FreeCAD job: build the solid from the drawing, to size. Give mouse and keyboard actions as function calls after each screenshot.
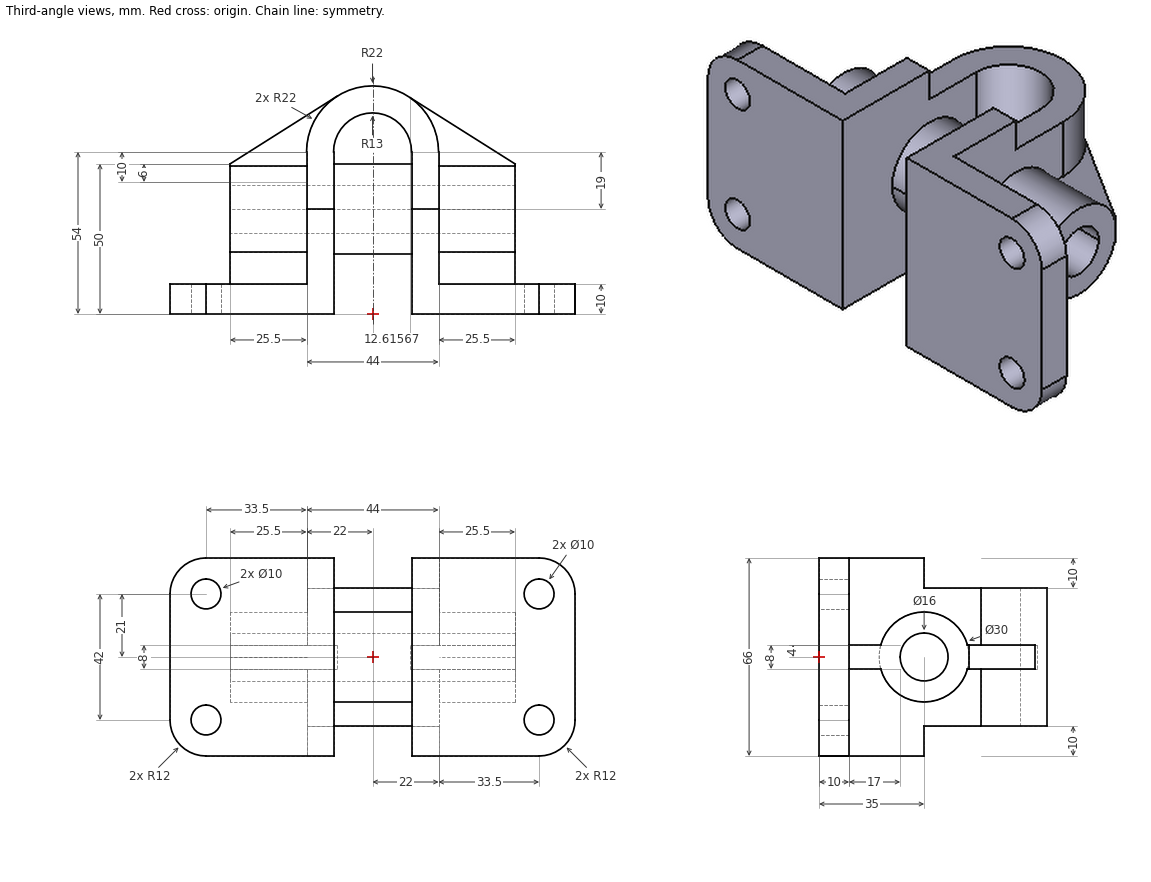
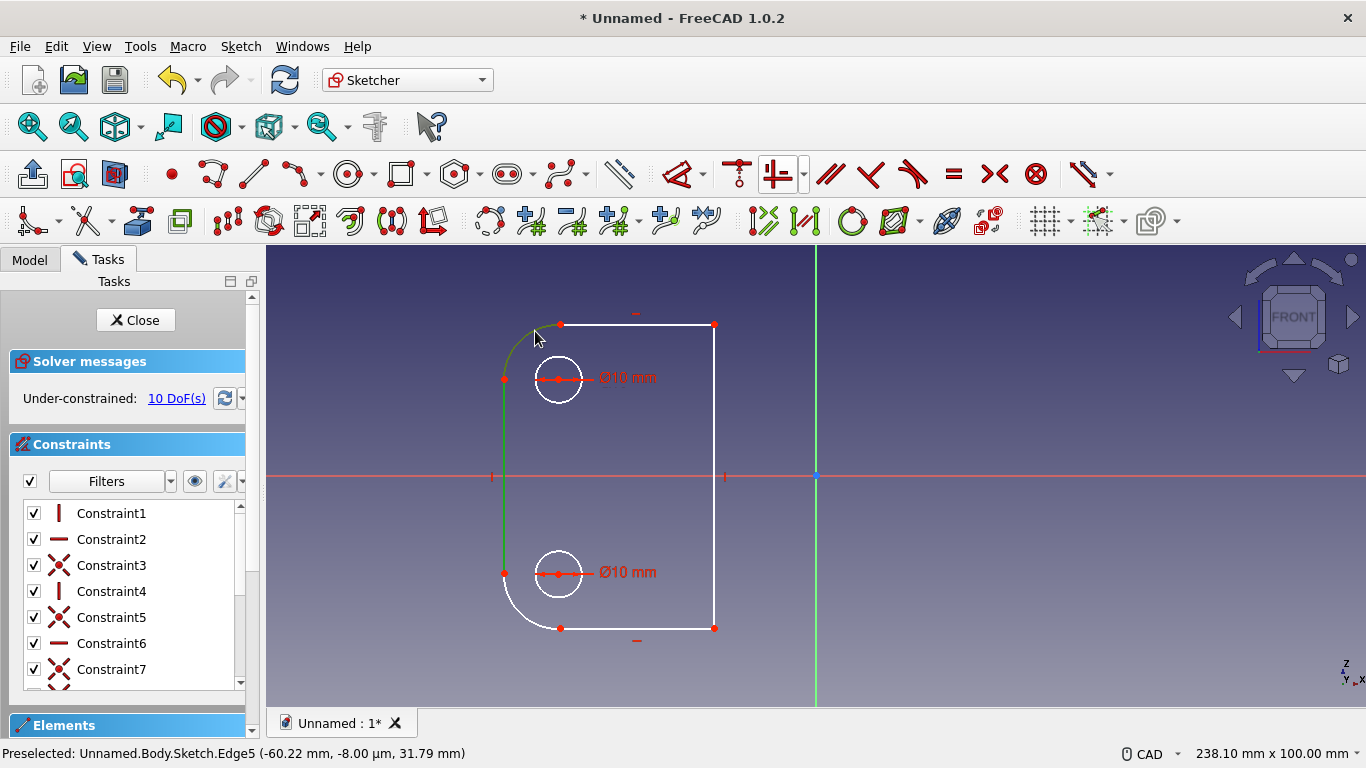
click(913, 174)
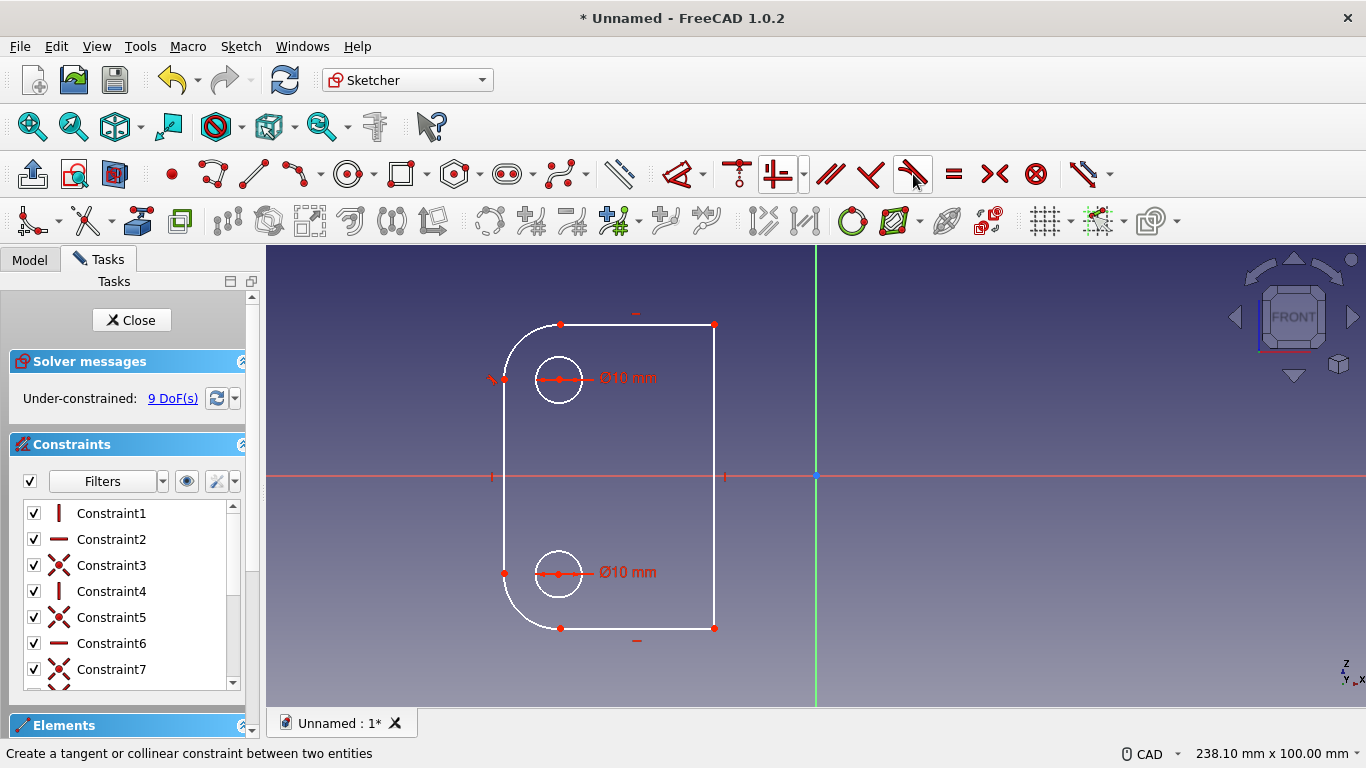
click(504, 516)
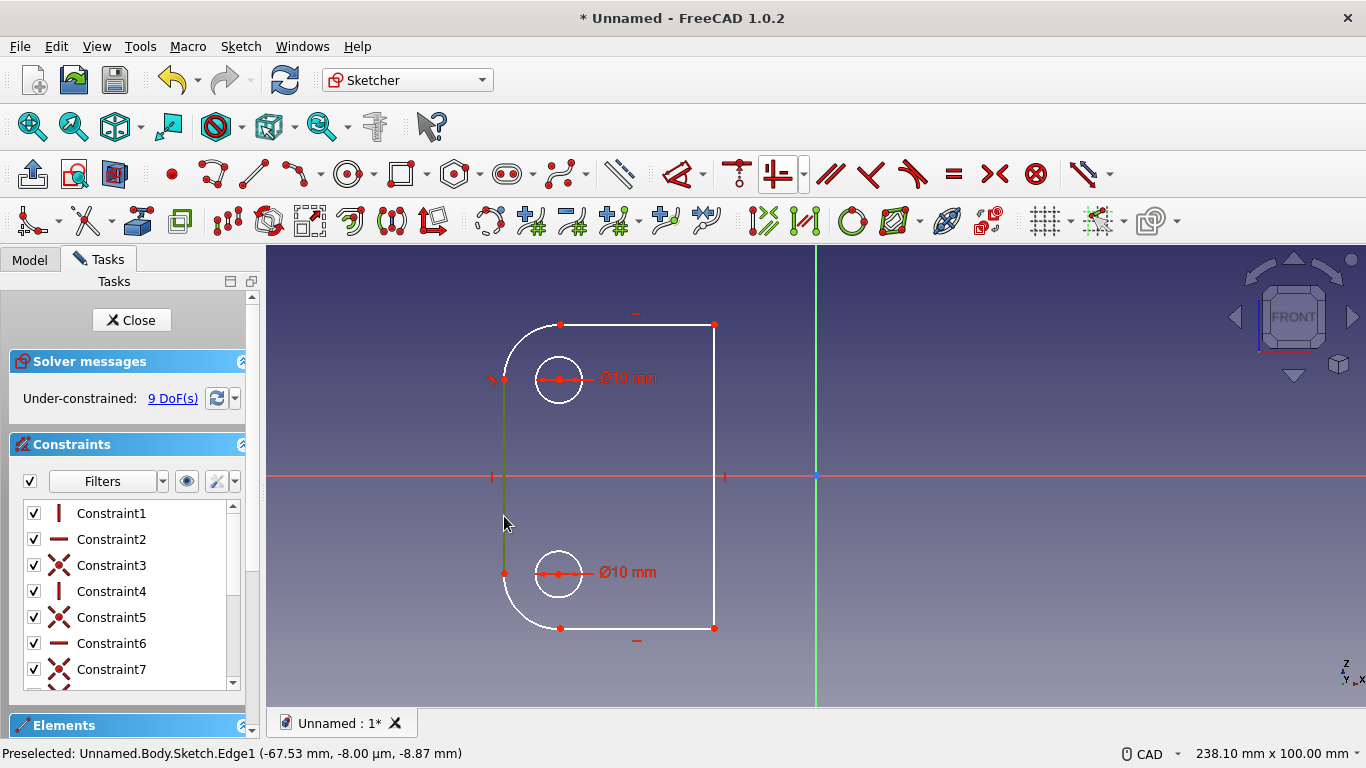
click(510, 599)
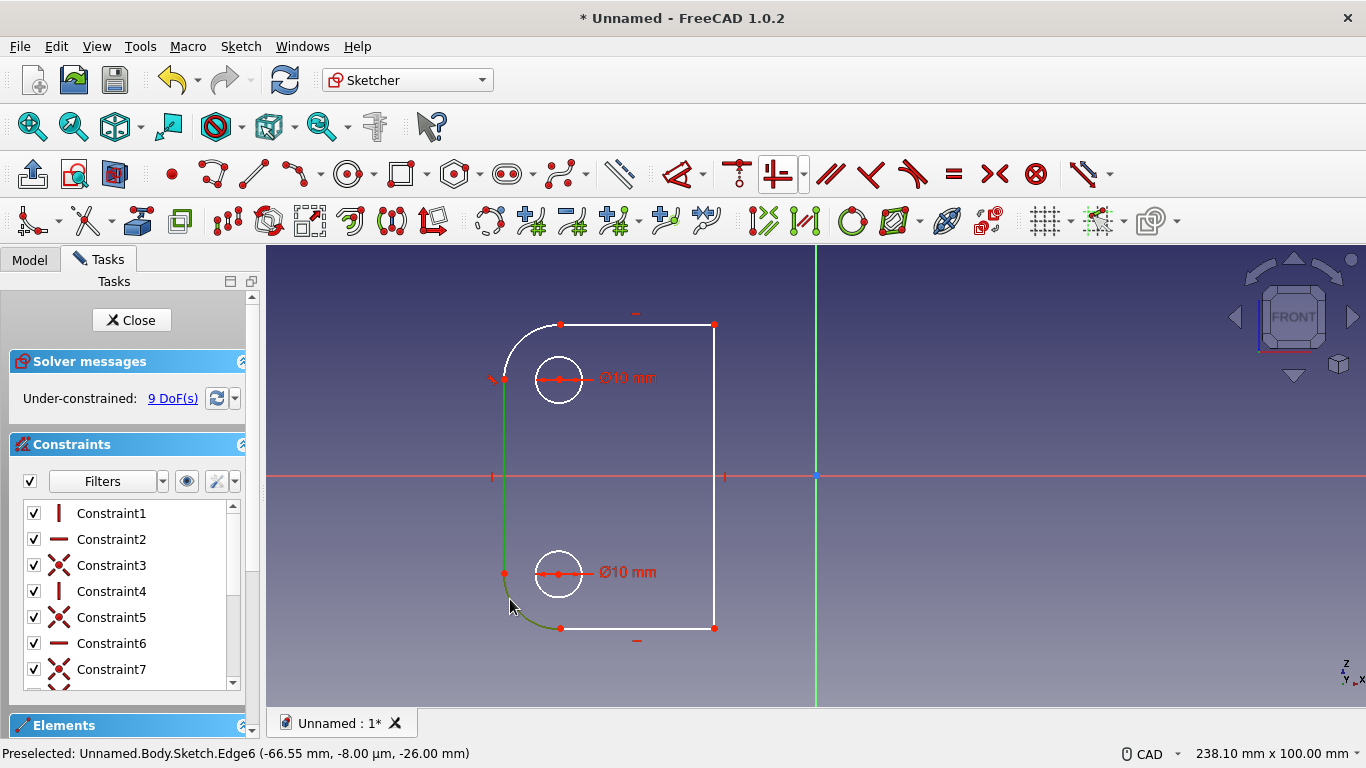
click(913, 174)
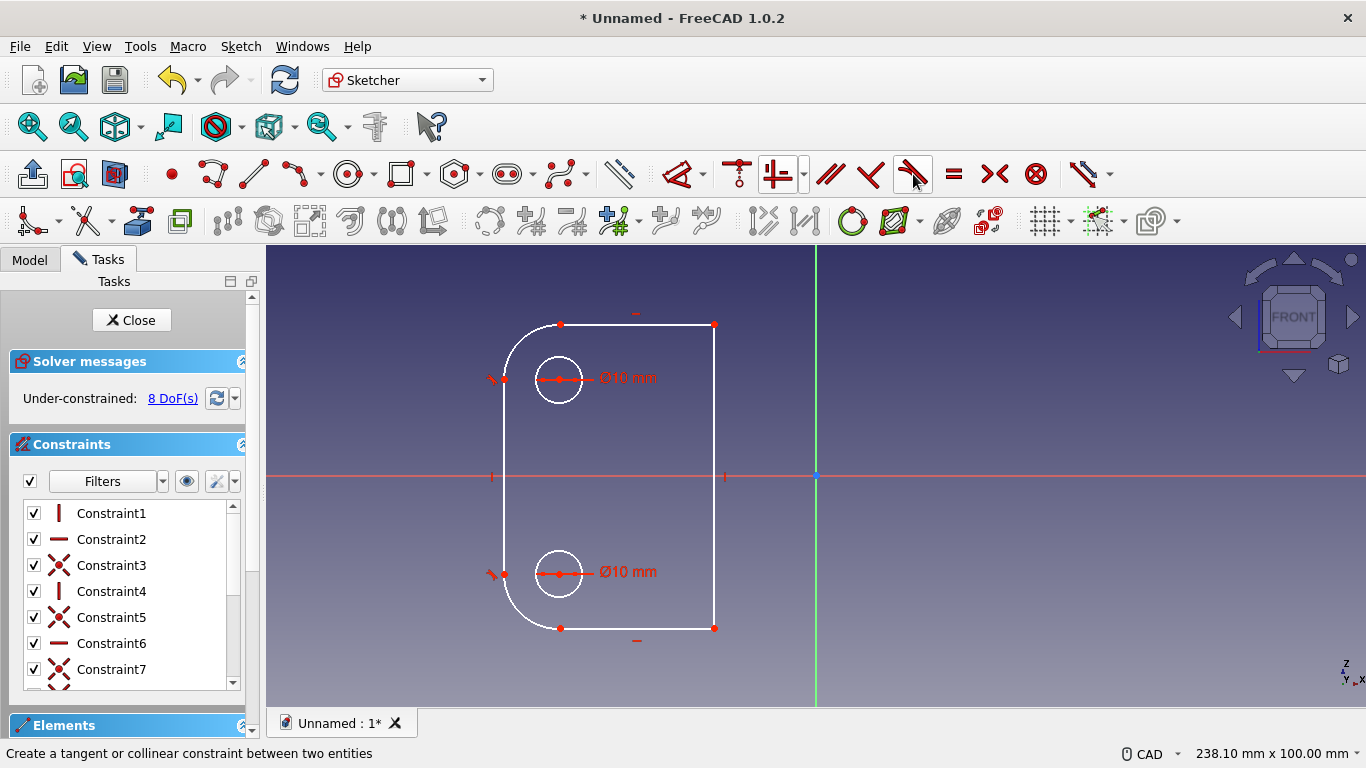
click(606, 325)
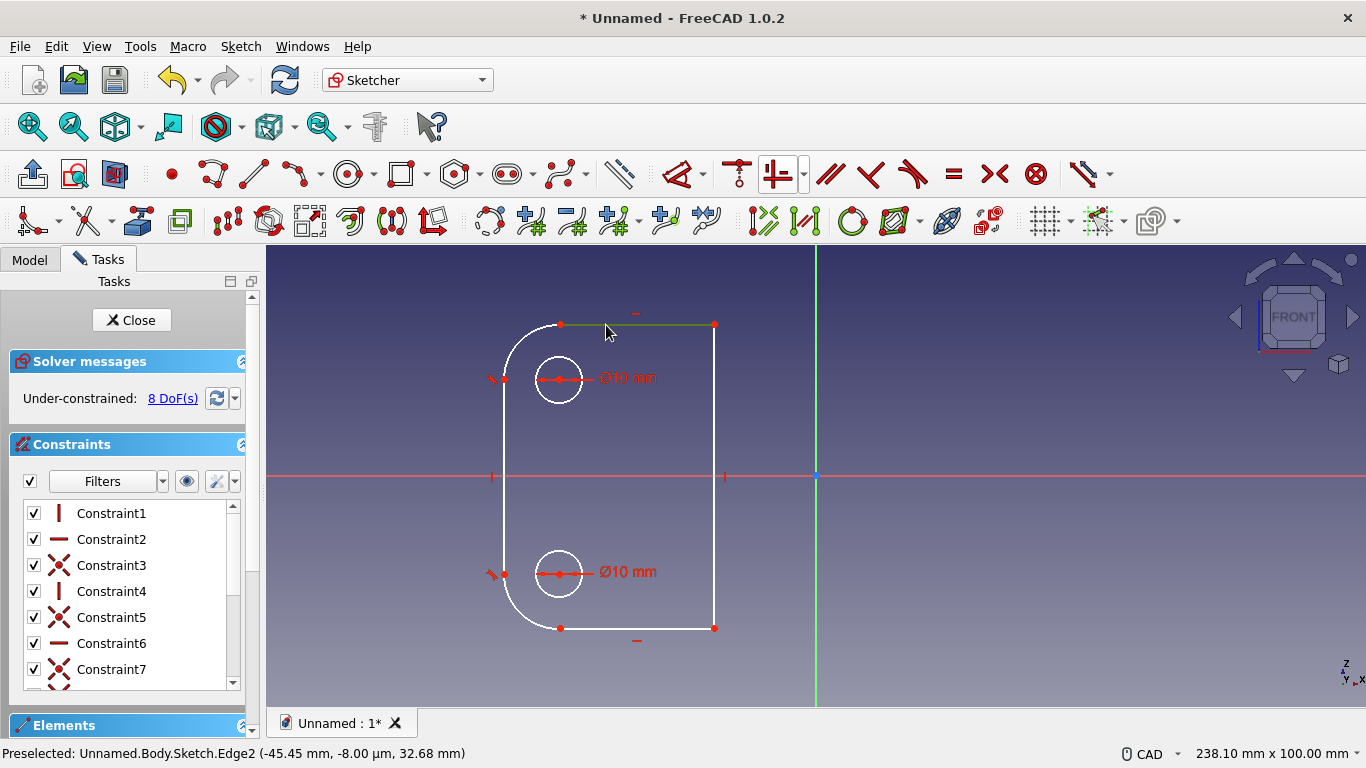
click(535, 331)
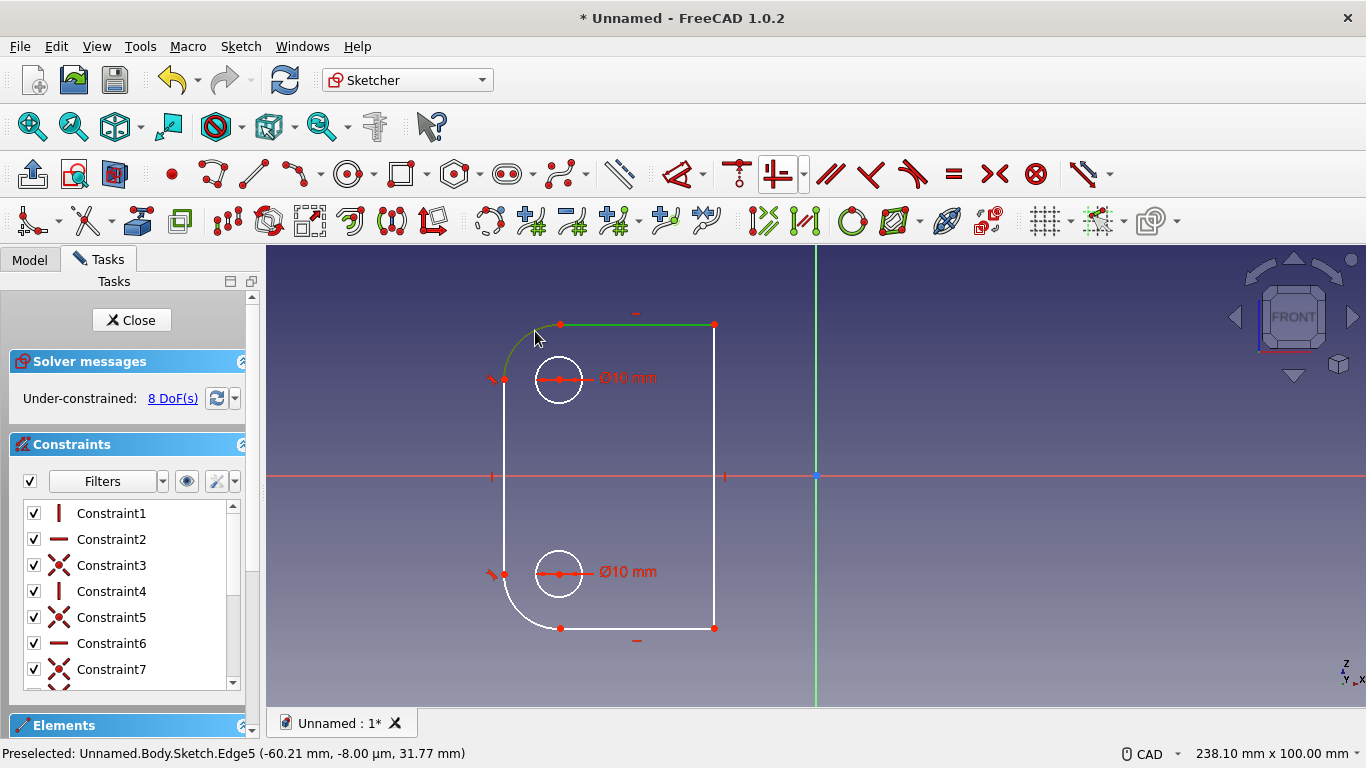
click(913, 174)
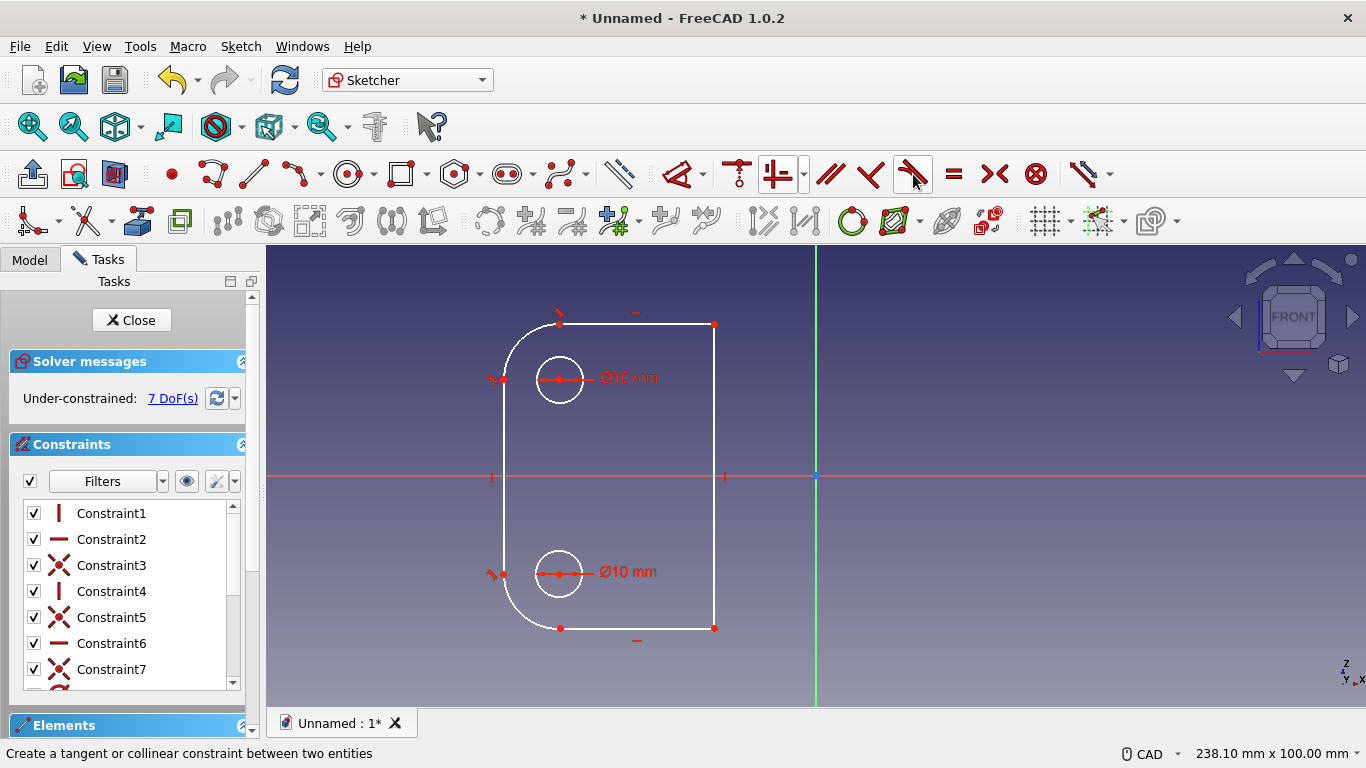
click(668, 629)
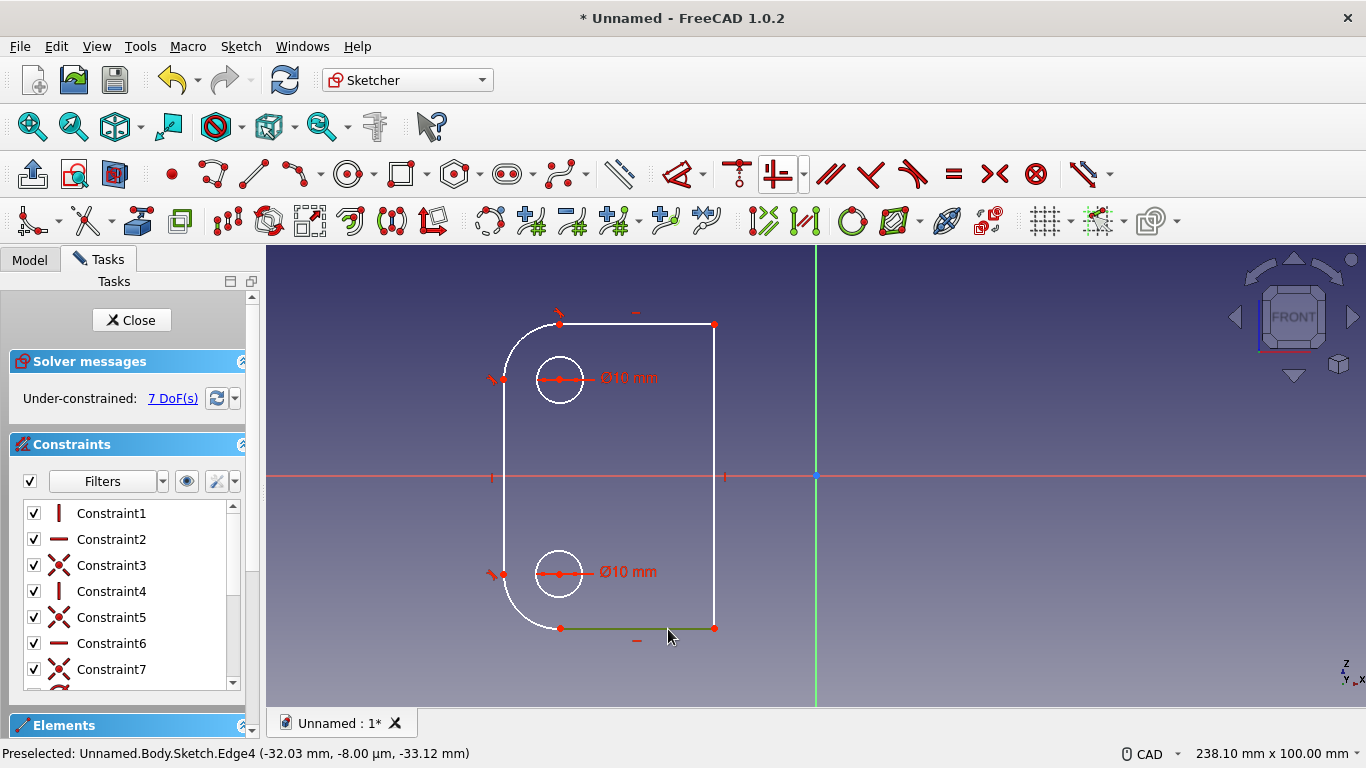
click(510, 599)